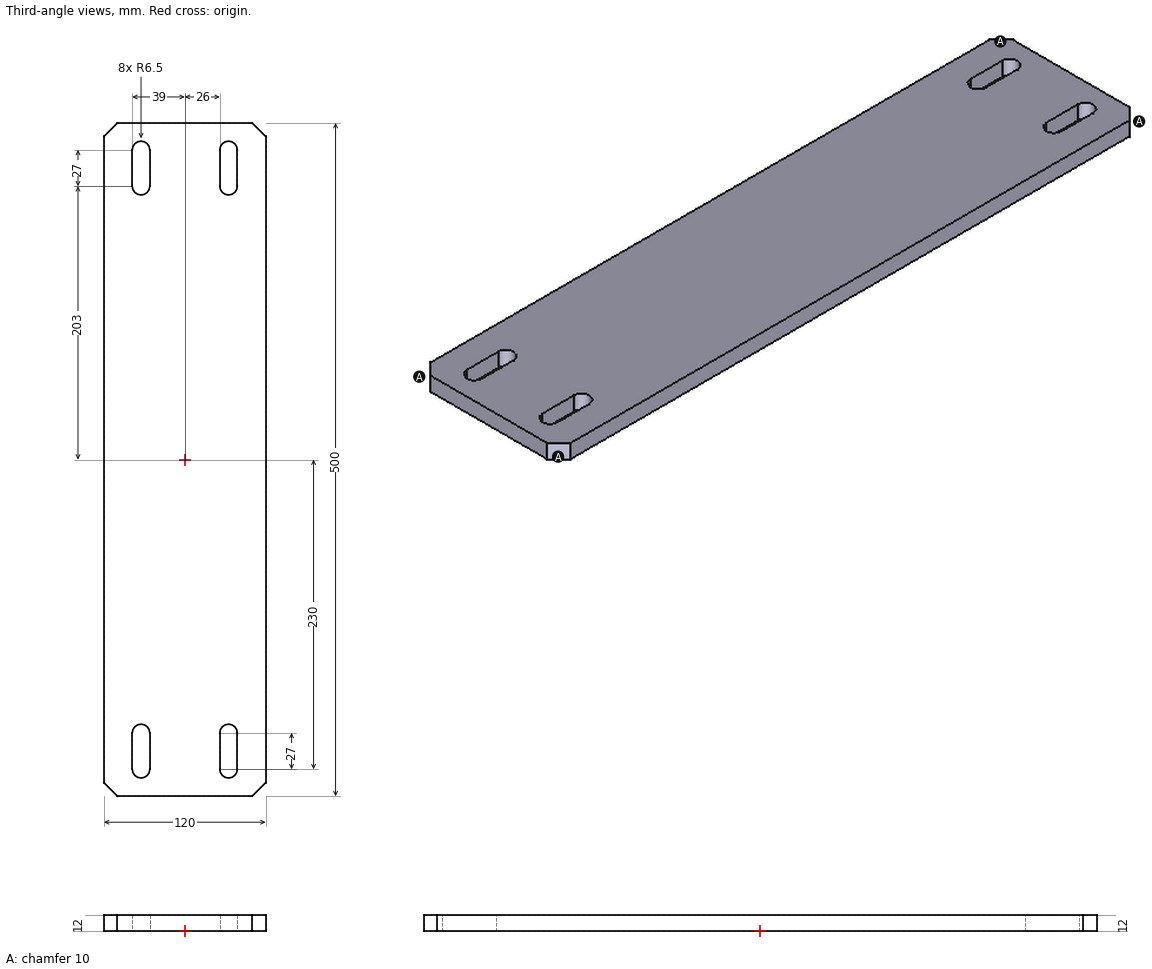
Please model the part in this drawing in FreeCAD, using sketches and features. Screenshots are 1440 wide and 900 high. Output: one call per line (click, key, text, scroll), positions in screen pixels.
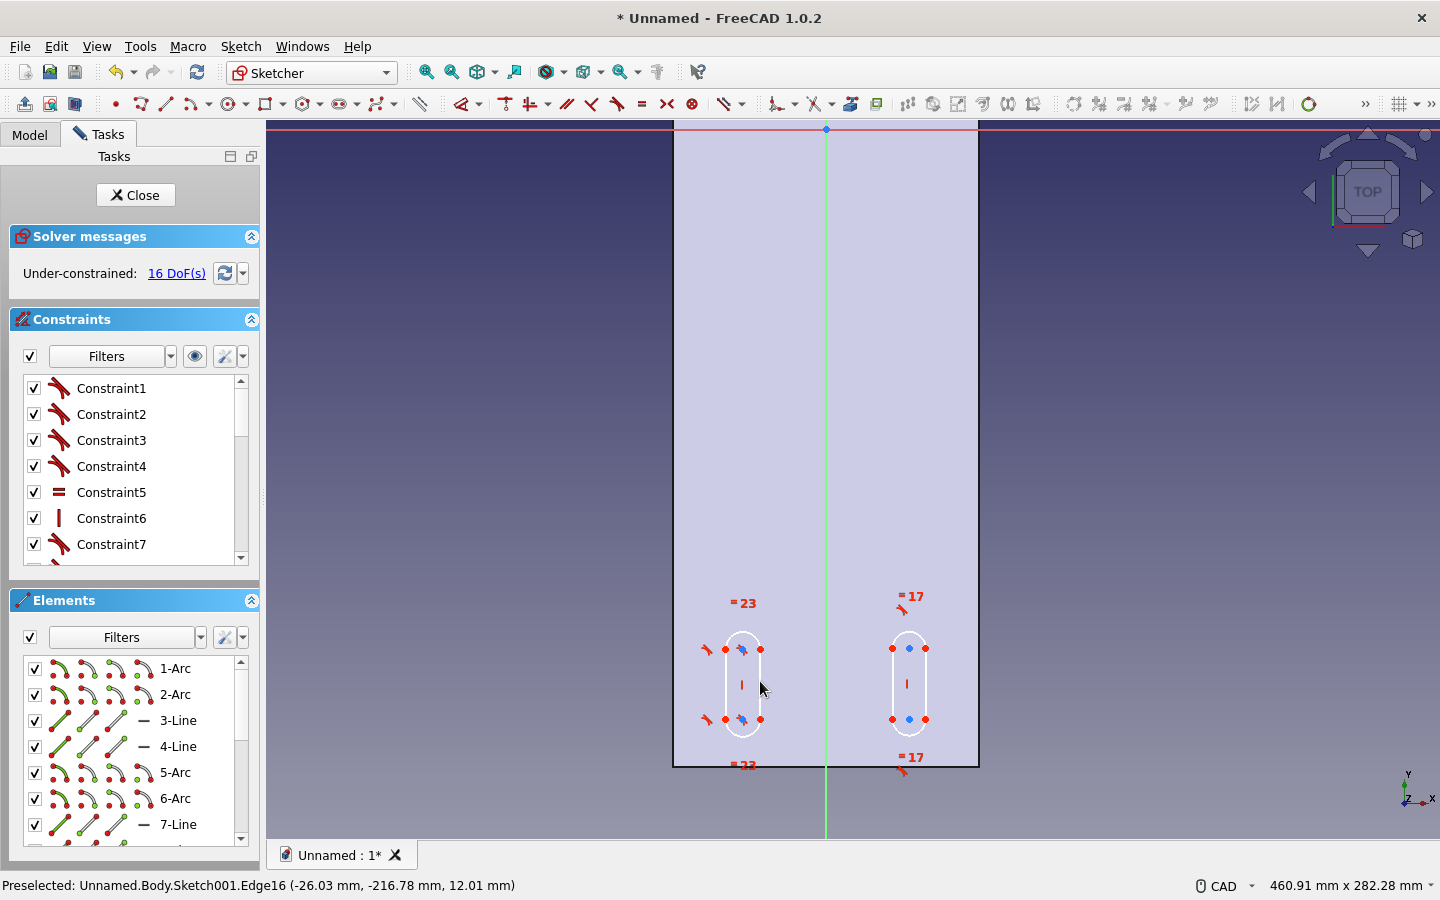
scroll(760, 683, down, 5)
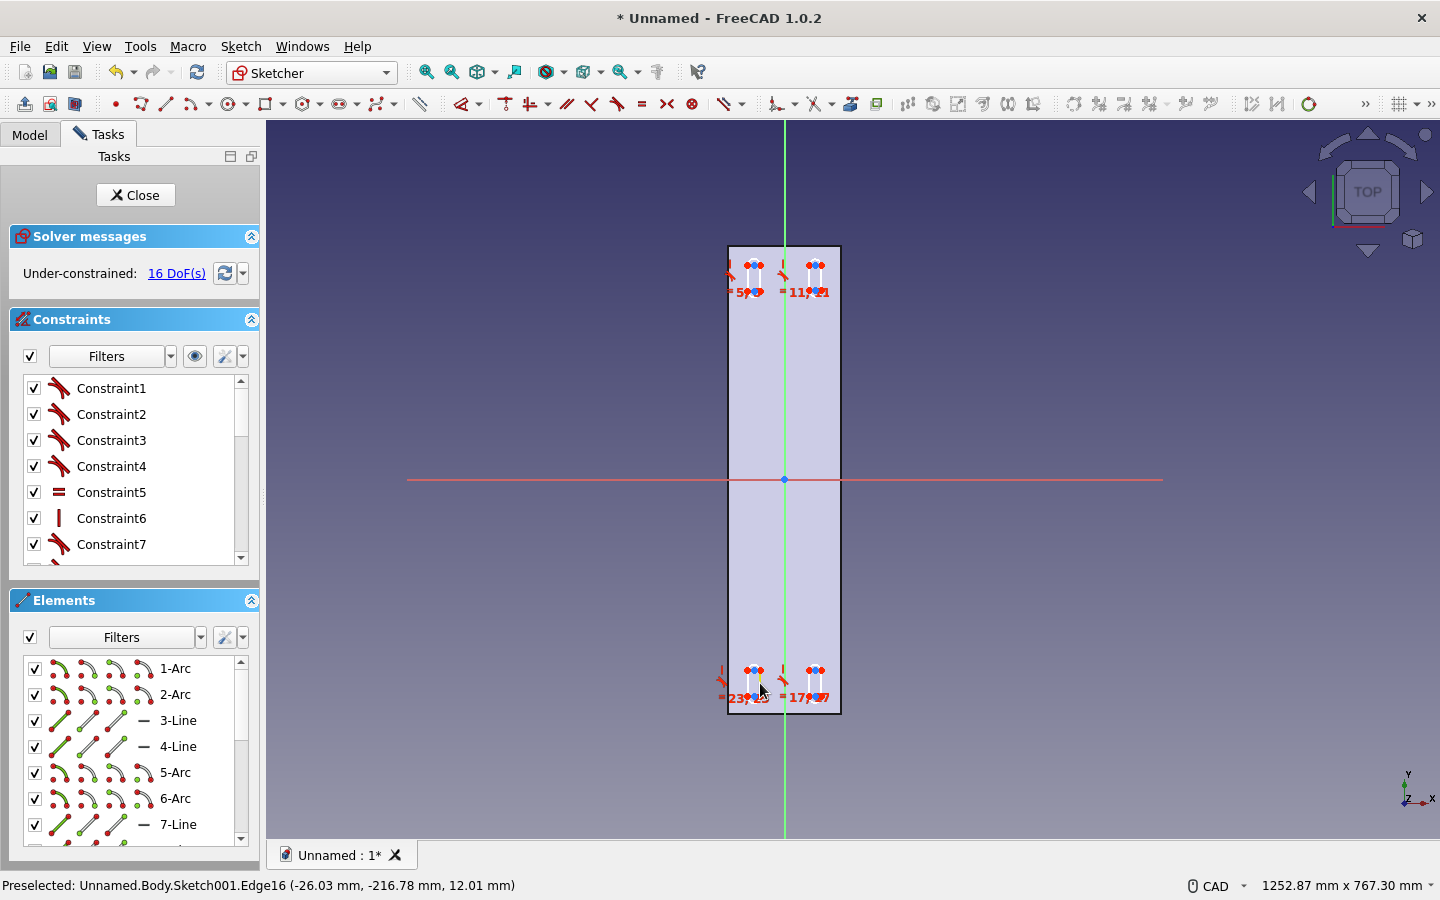
scroll(750, 296, up, 5)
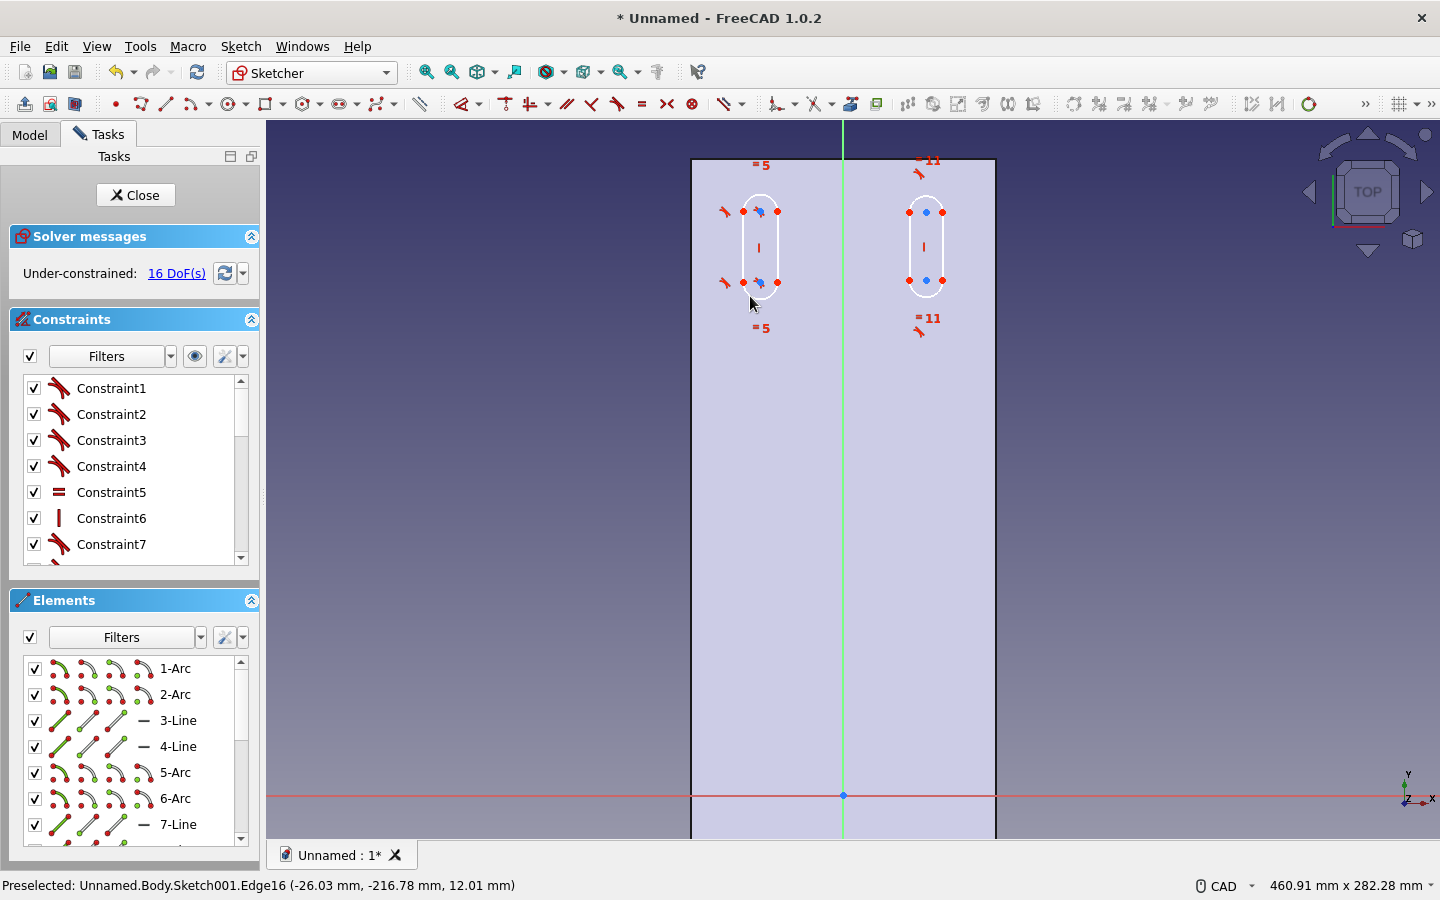
click(750, 296)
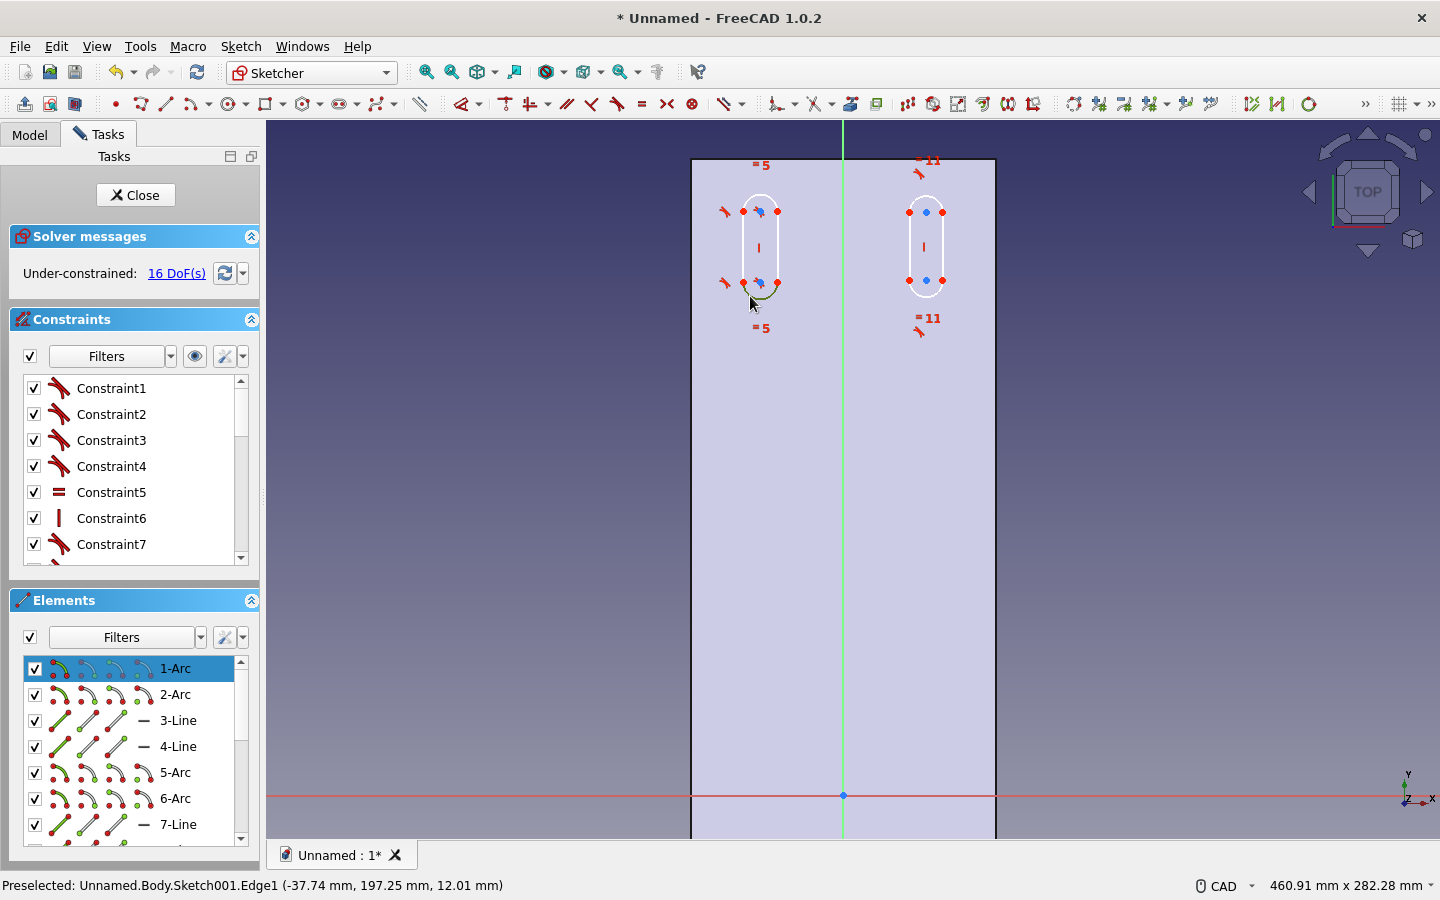
click(917, 294)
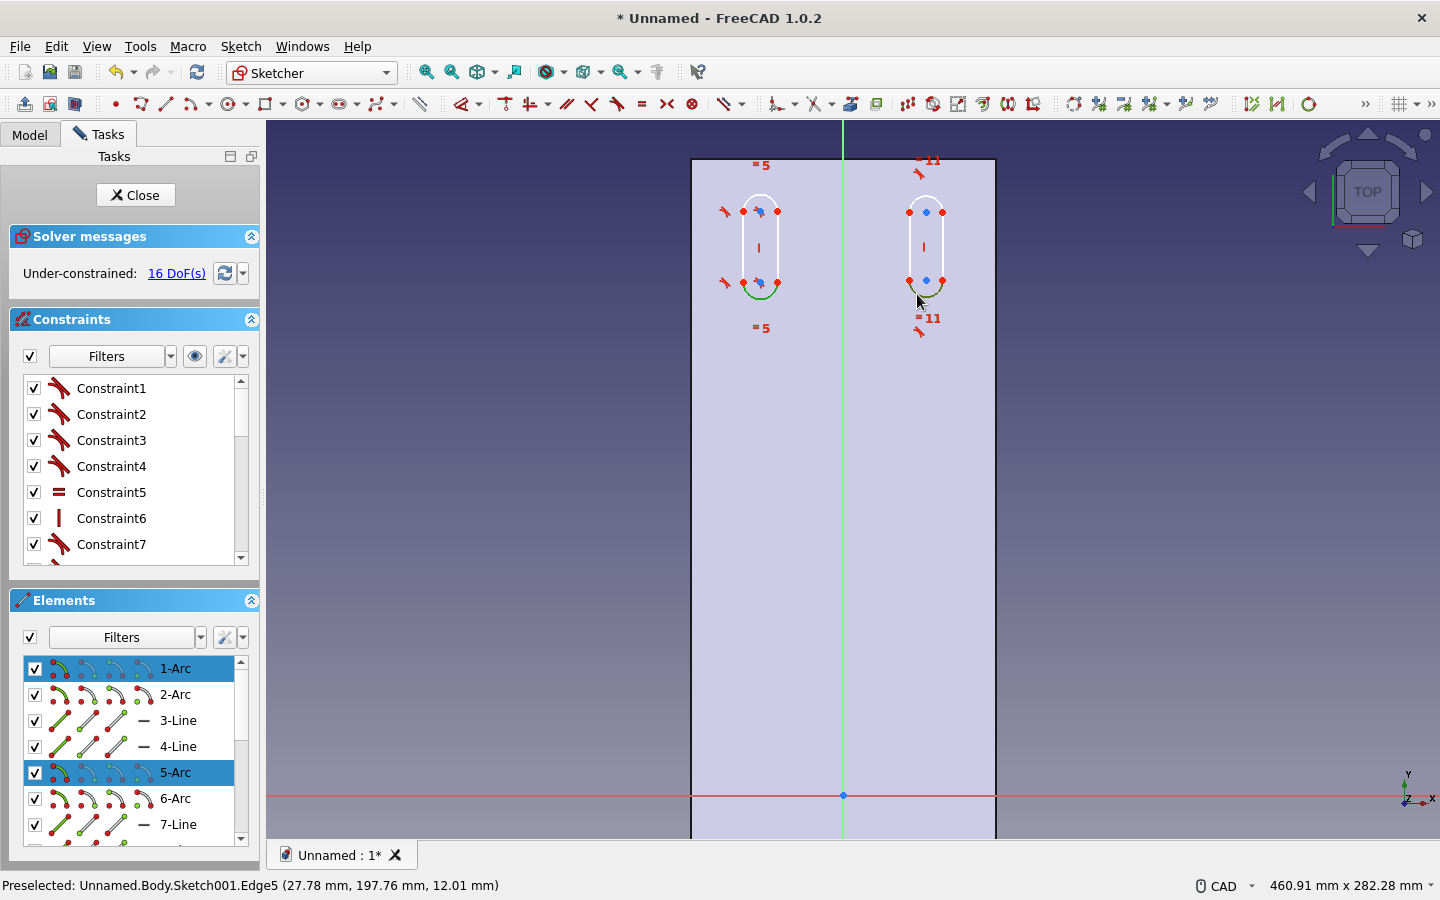
scroll(750, 295, down, 5)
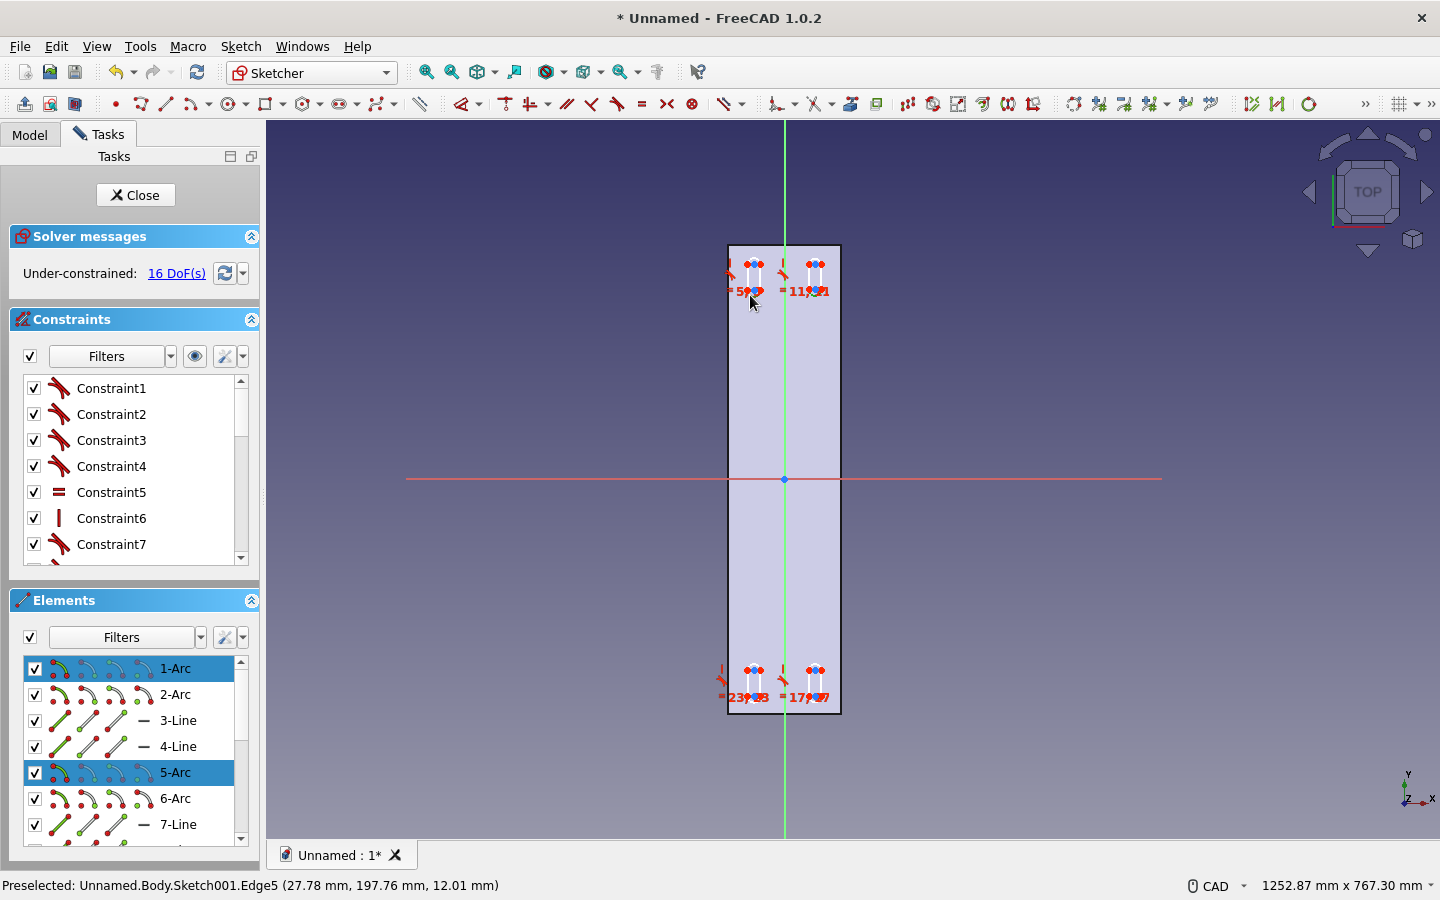
scroll(812, 701, up, 5)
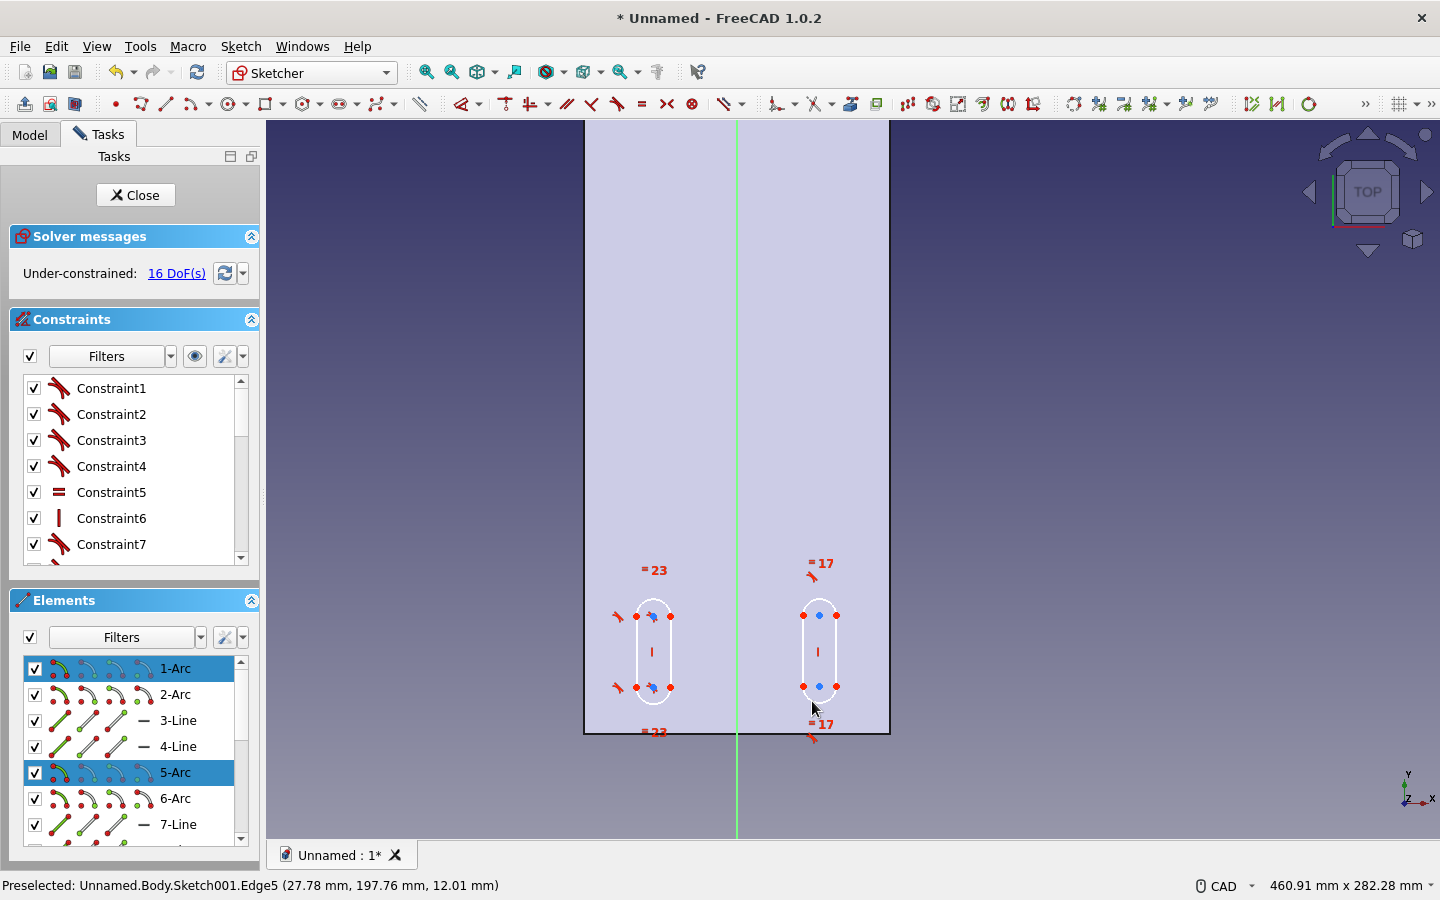
click(810, 700)